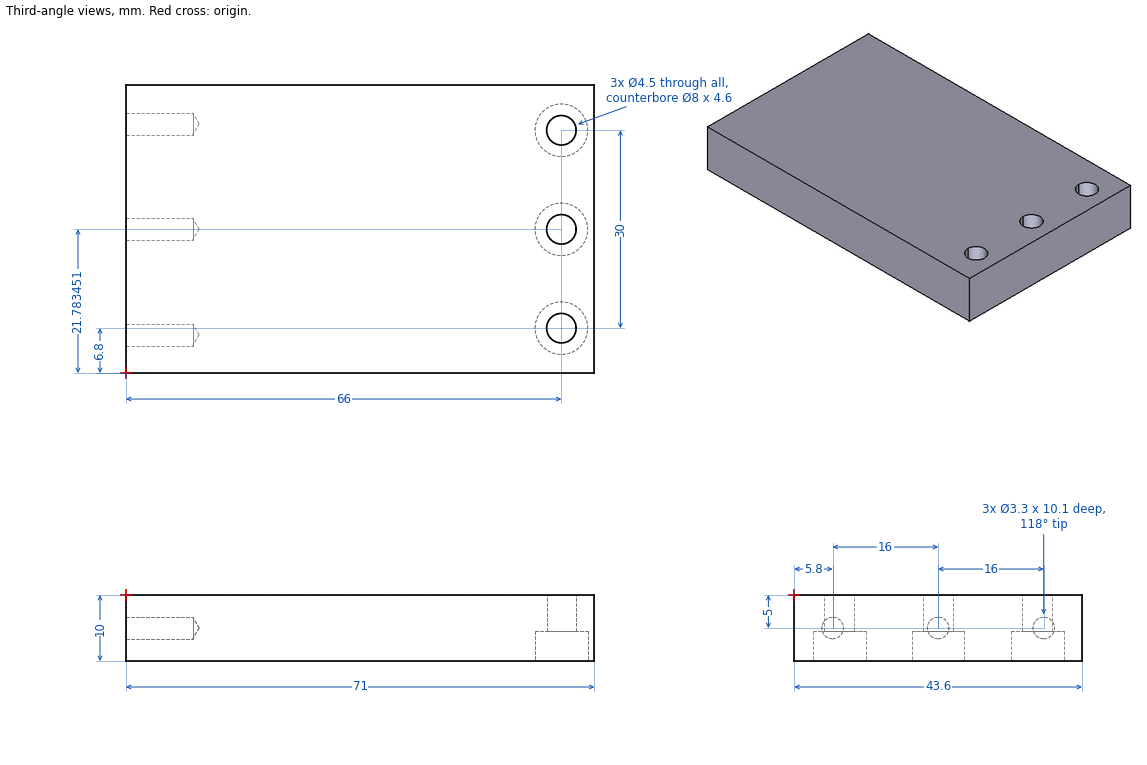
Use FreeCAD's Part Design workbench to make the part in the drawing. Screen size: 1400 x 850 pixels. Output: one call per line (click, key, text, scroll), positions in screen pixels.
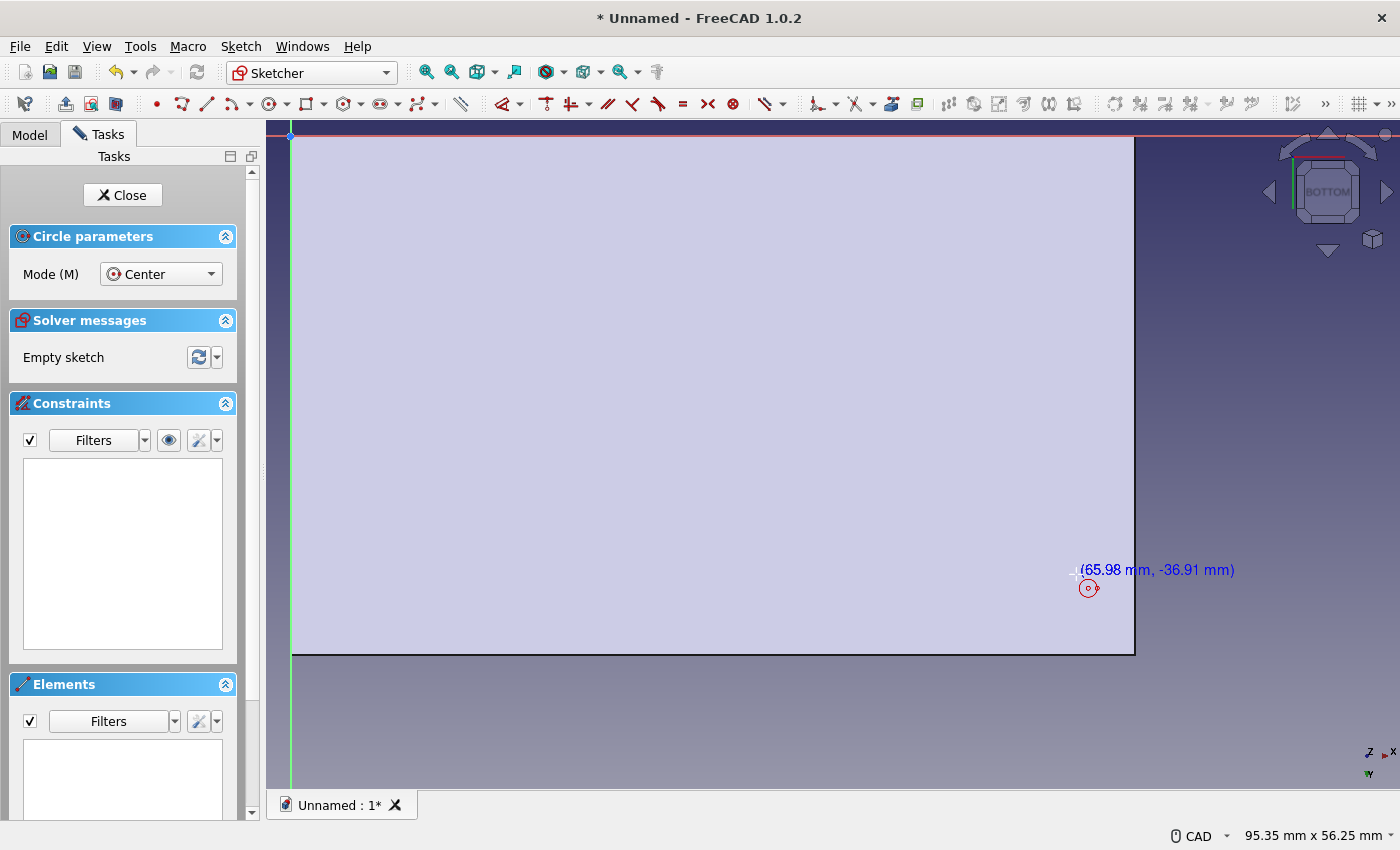
click(1076, 574)
click(1095, 555)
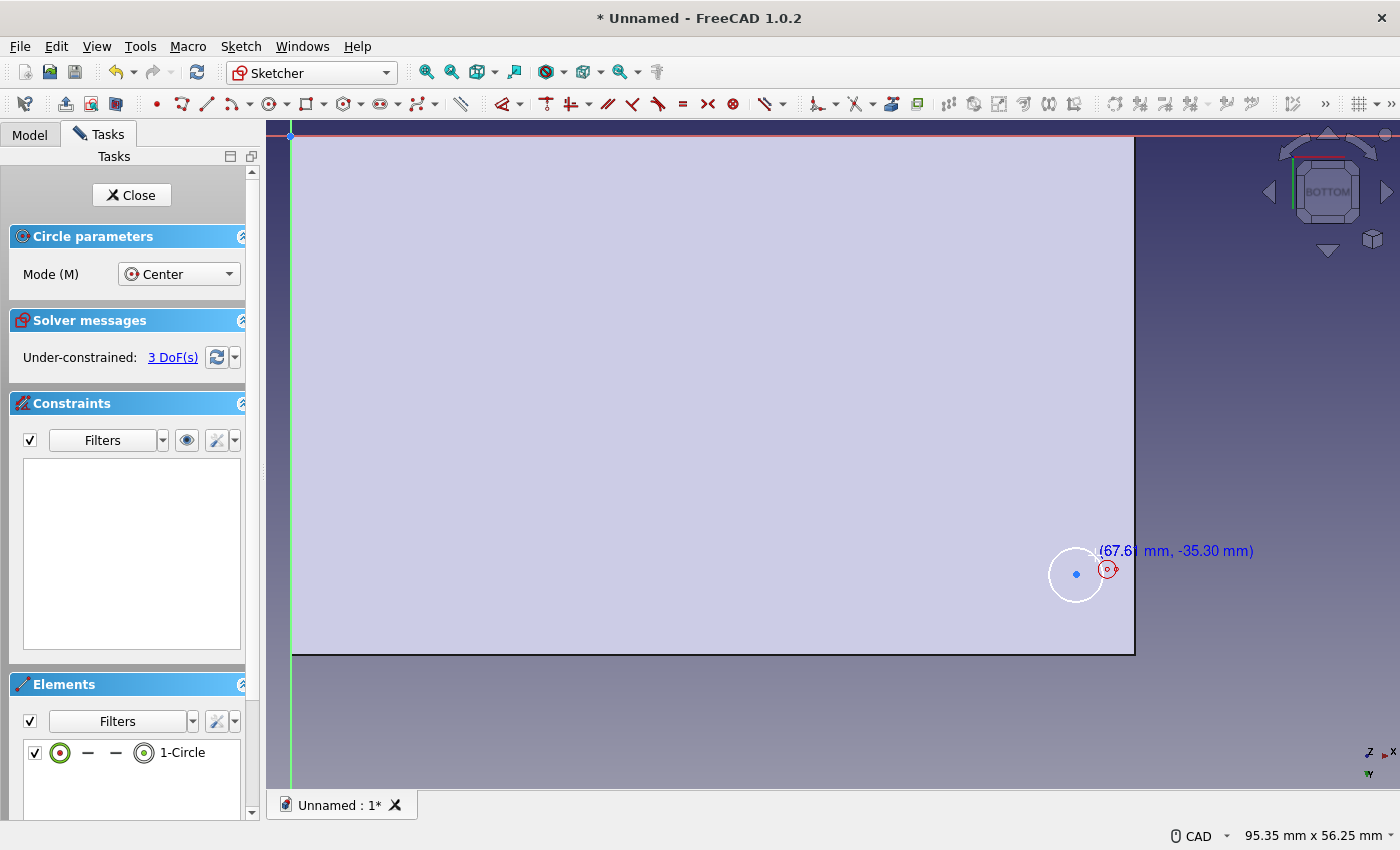
click(1076, 395)
click(1095, 376)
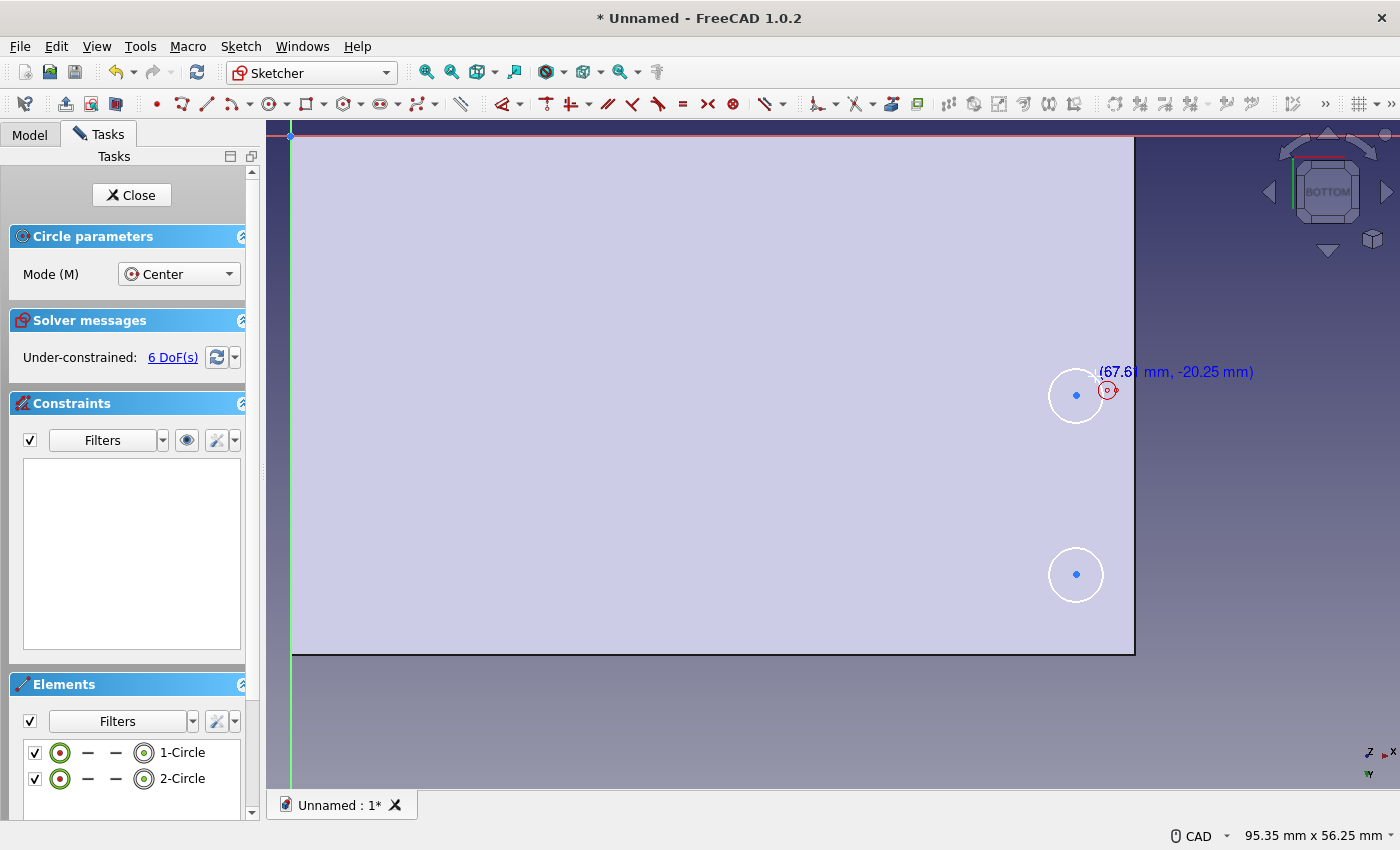
click(1076, 217)
click(1095, 198)
key(Escape)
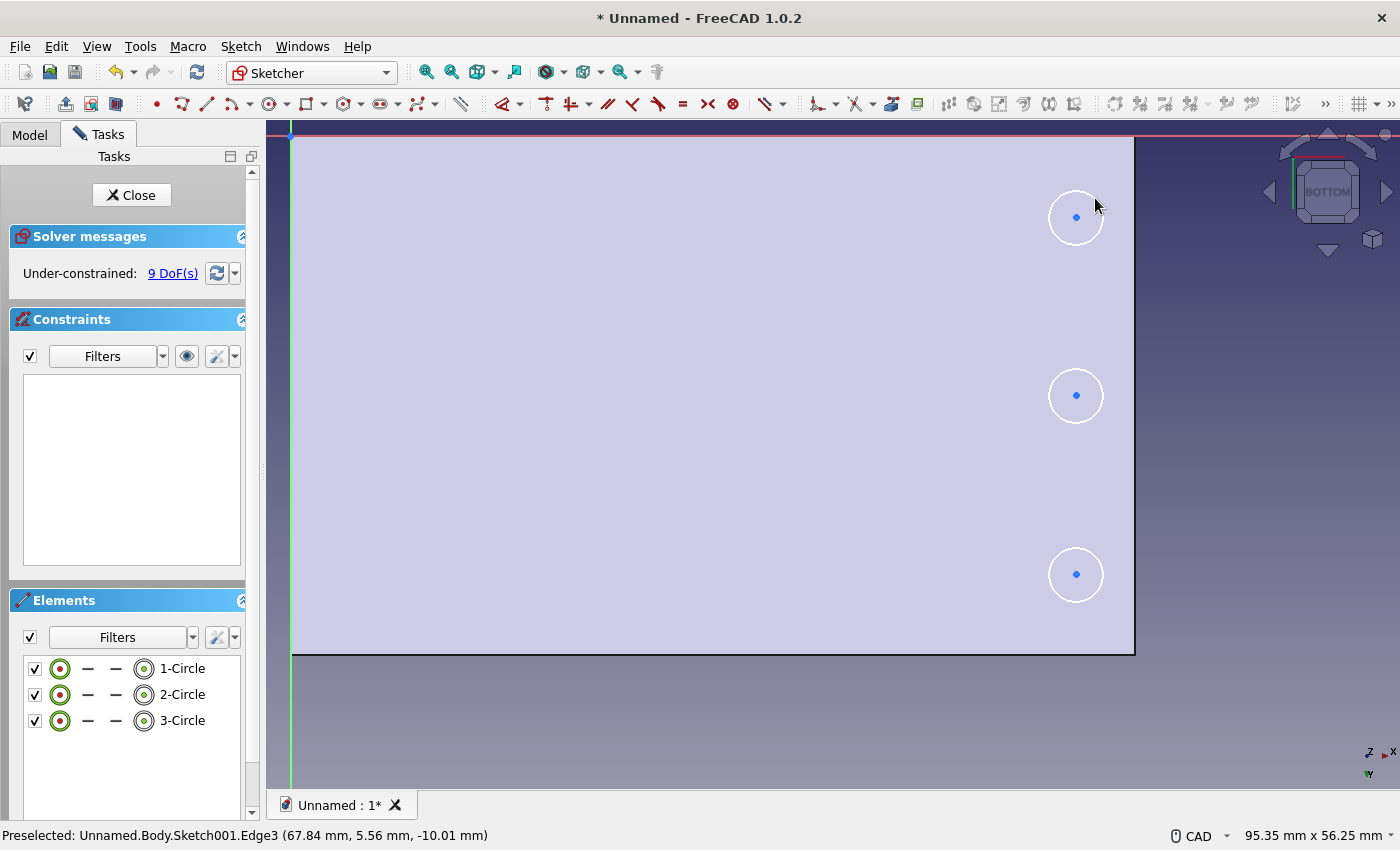
click(1095, 556)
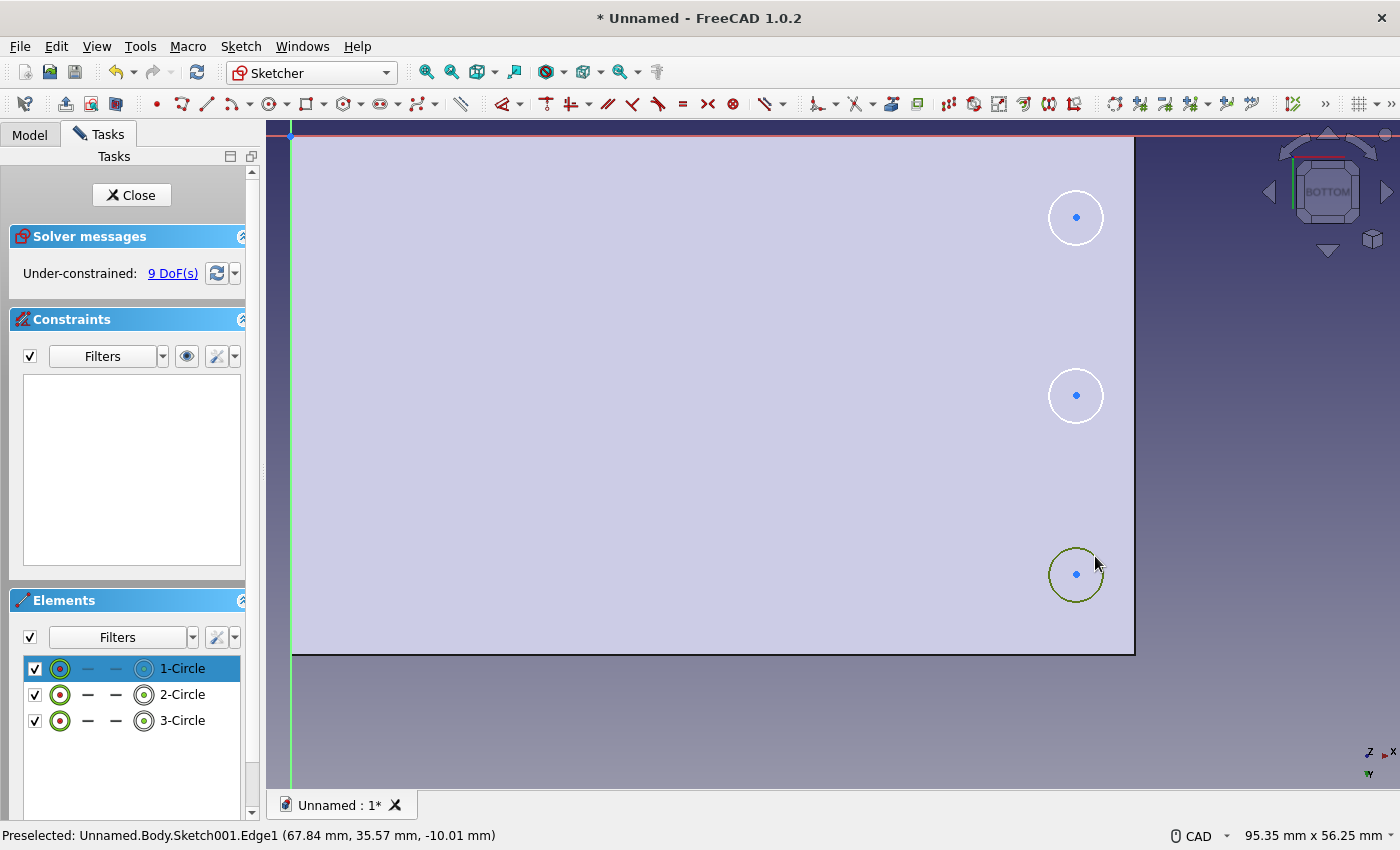
click(1095, 377)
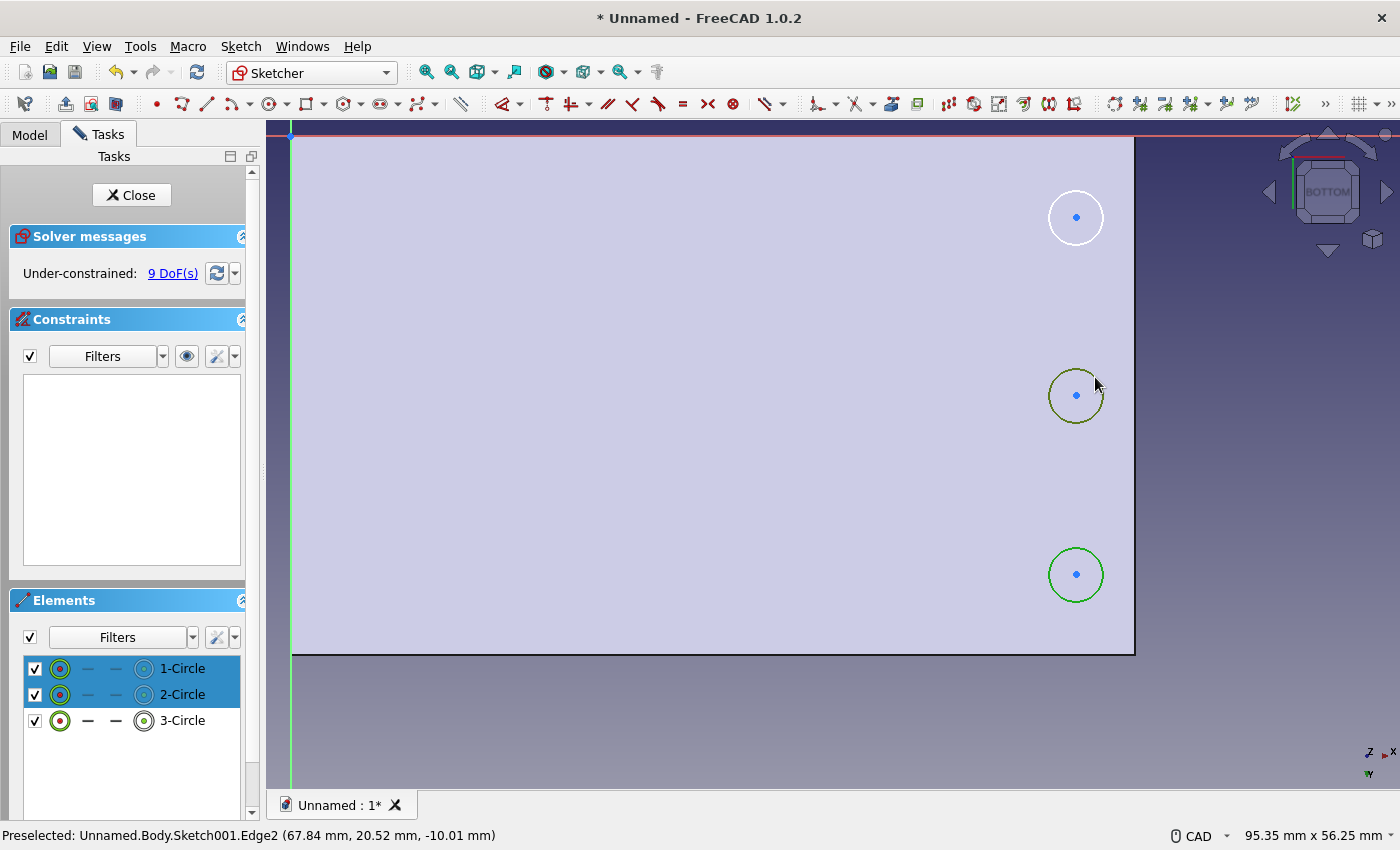
click(1095, 199)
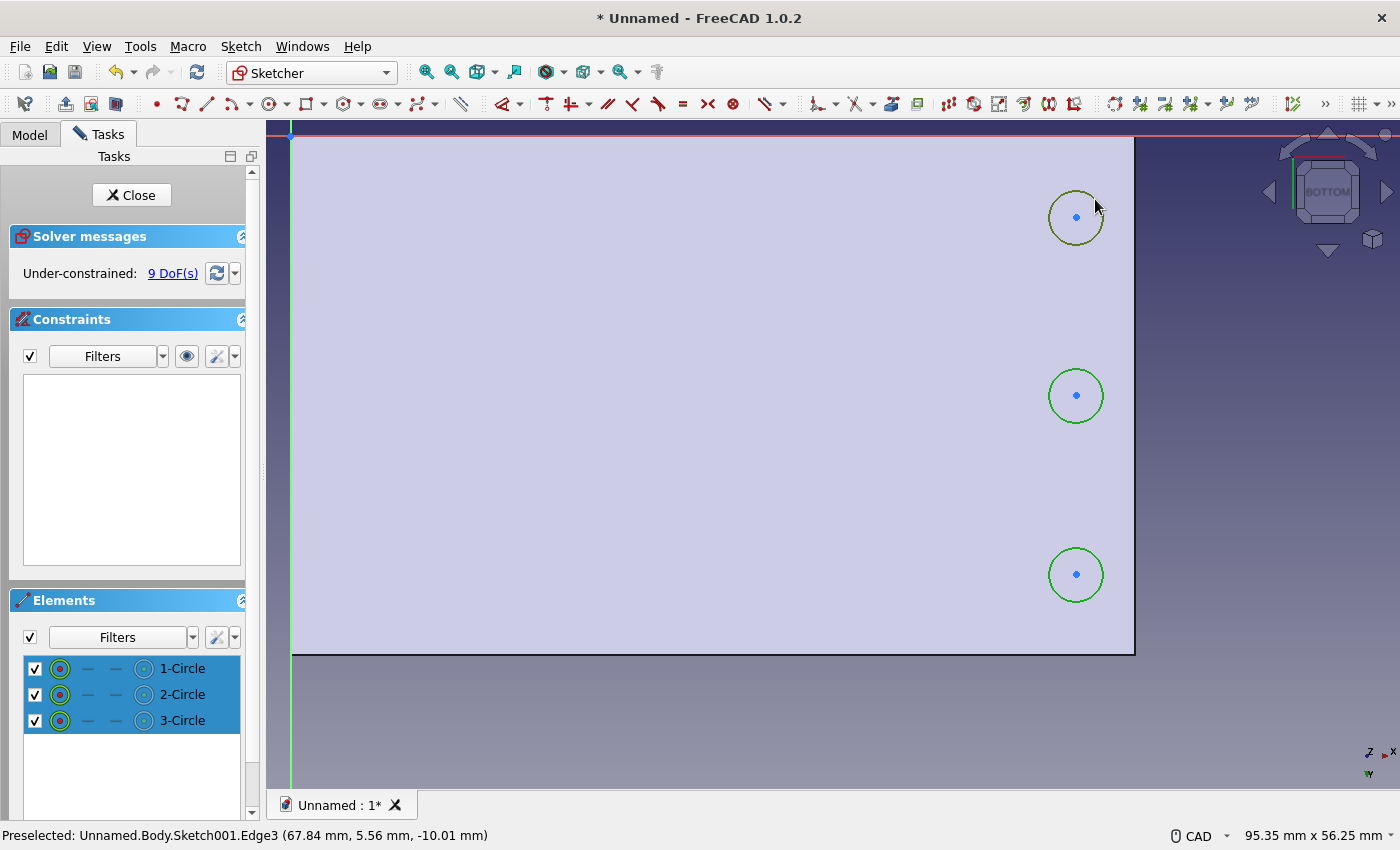
click(683, 104)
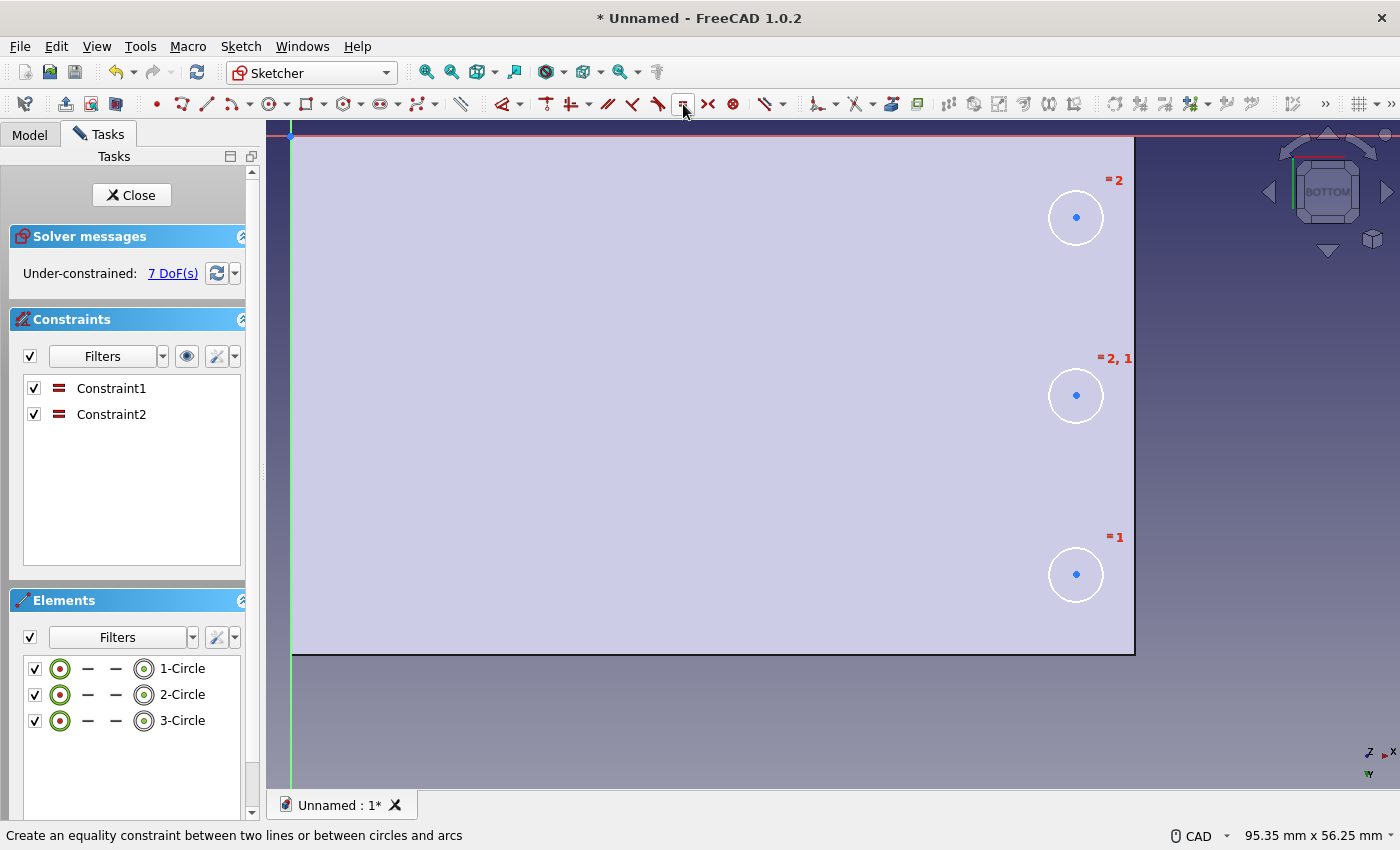
click(1076, 575)